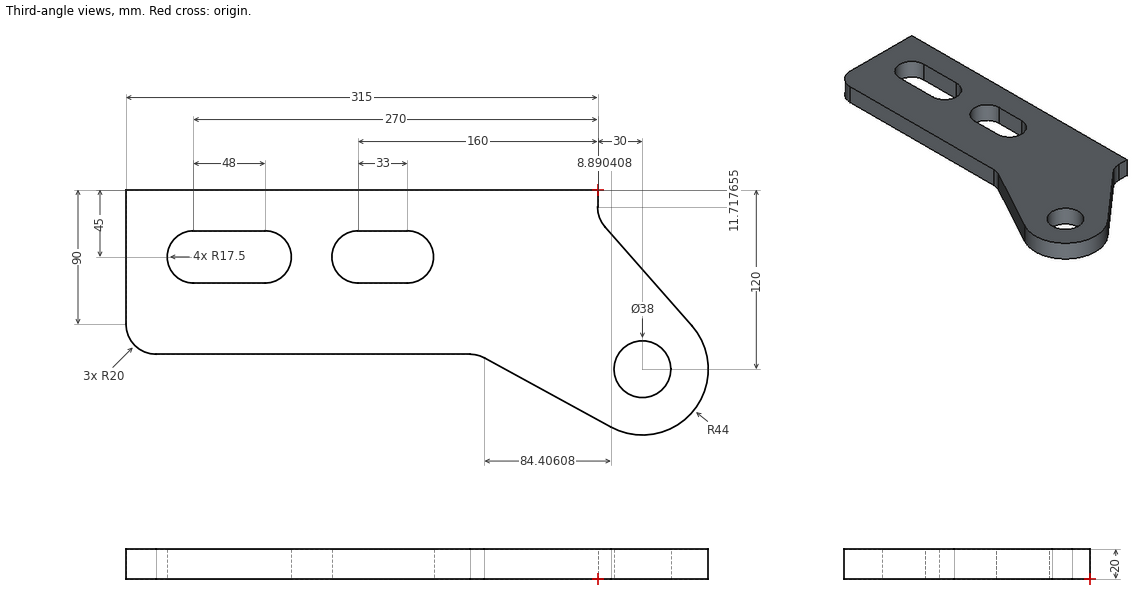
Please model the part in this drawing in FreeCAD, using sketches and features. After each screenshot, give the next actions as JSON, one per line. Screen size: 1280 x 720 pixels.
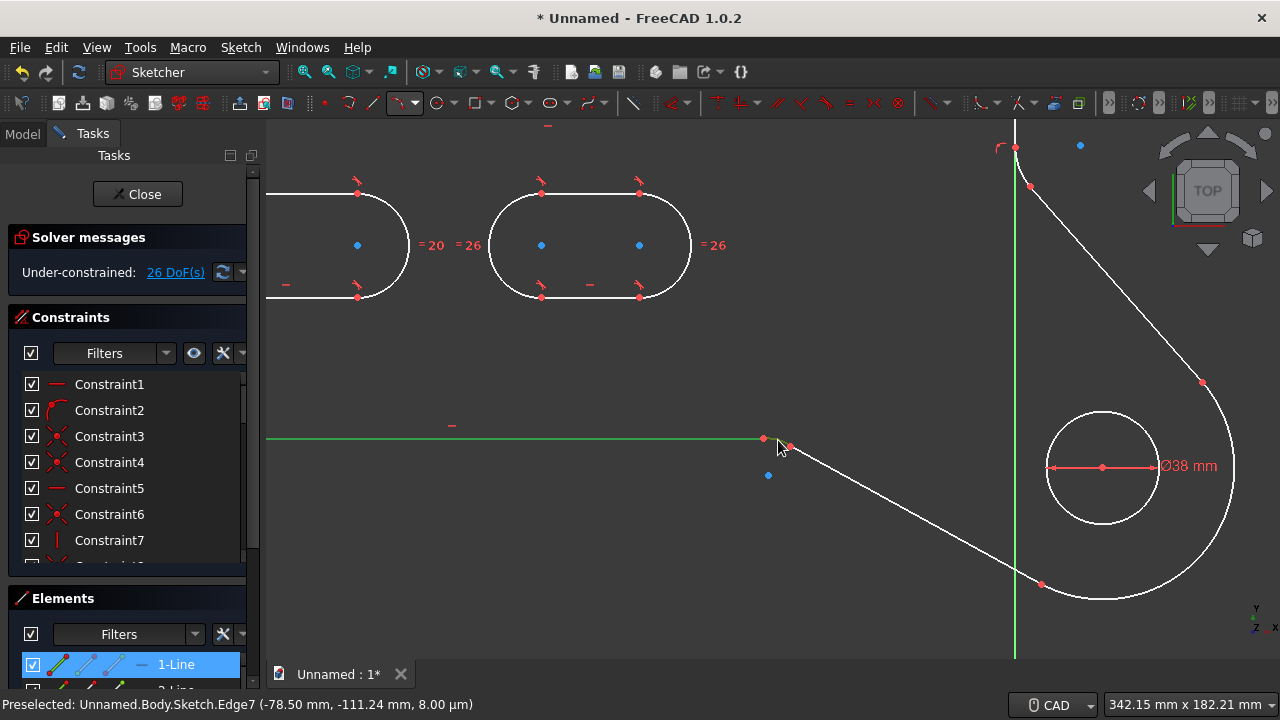
{"action": "left_click", "coordinate": [826, 104]}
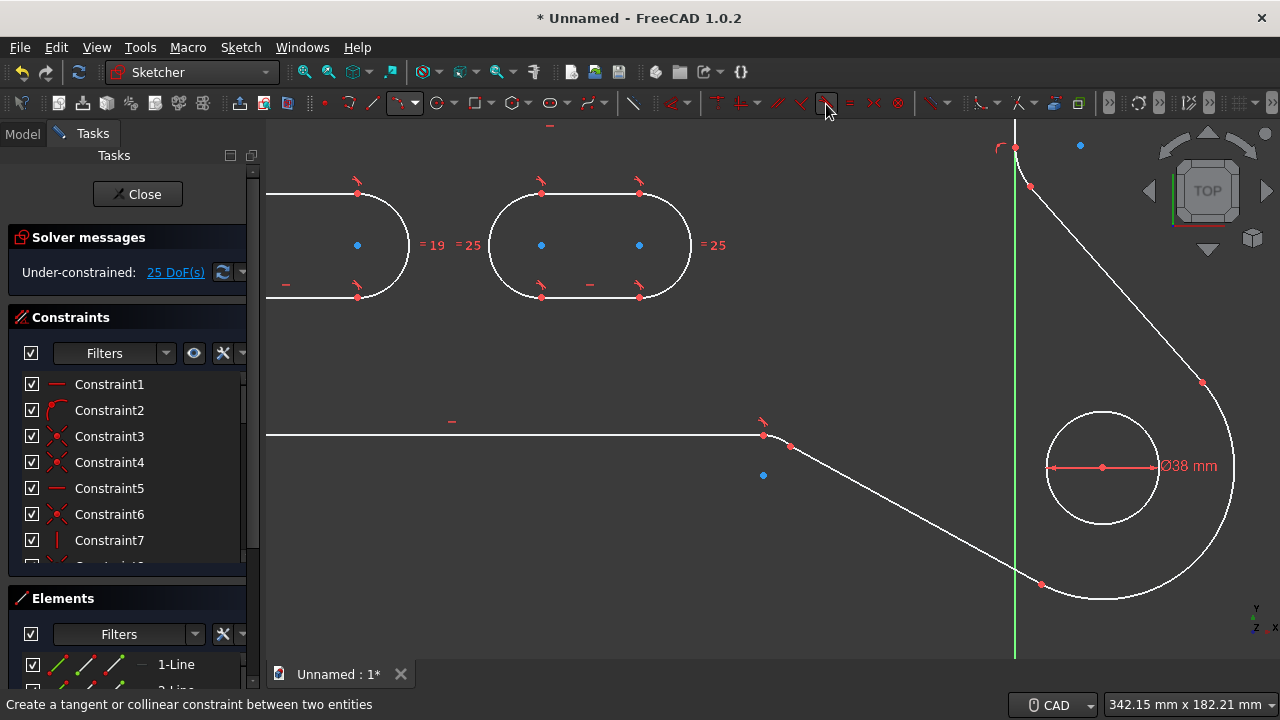
{"action": "left_click", "coordinate": [327, 435]}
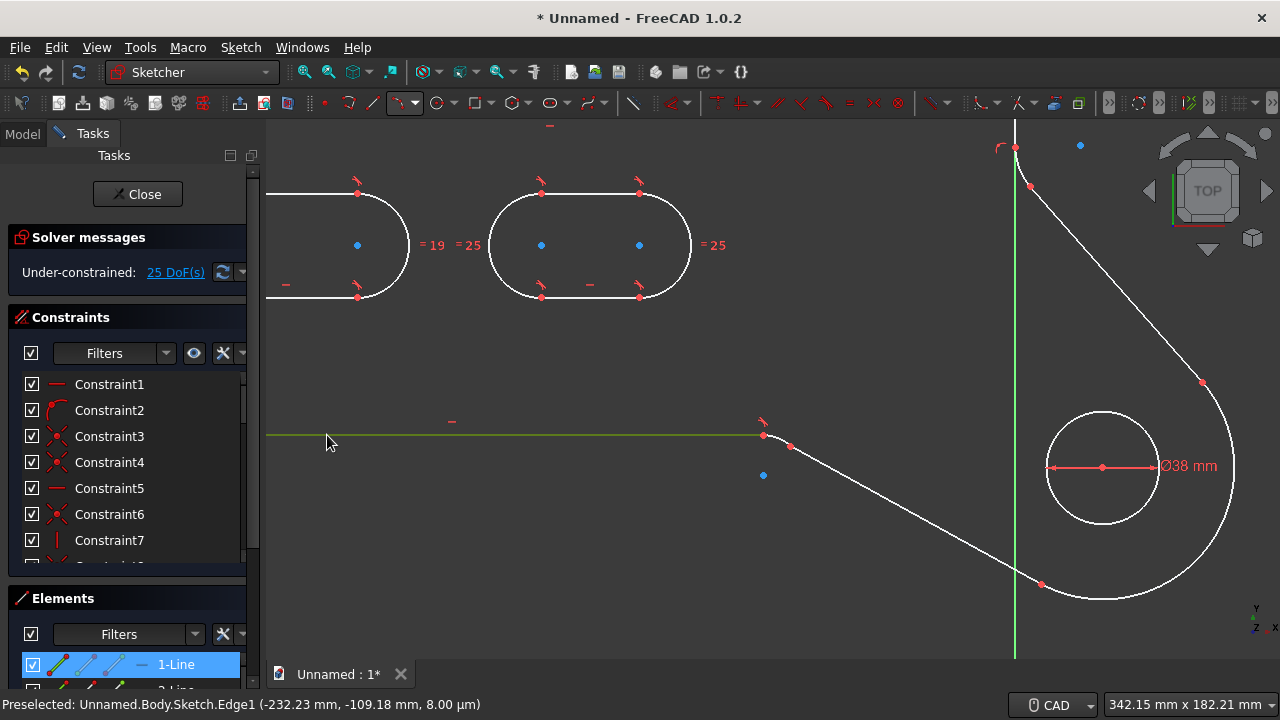
{"action": "scroll", "coordinate": [778, 440], "scroll_direction": "down", "scroll_amount": 3}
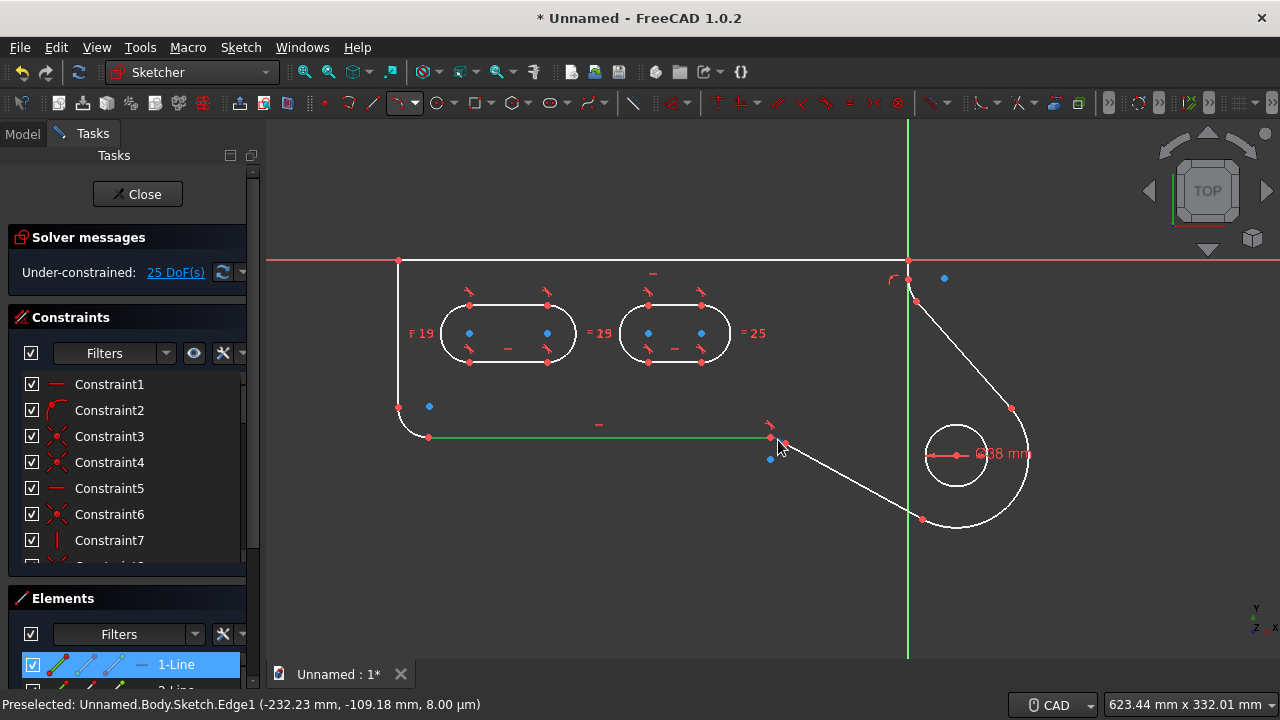
{"action": "left_click", "coordinate": [402, 421]}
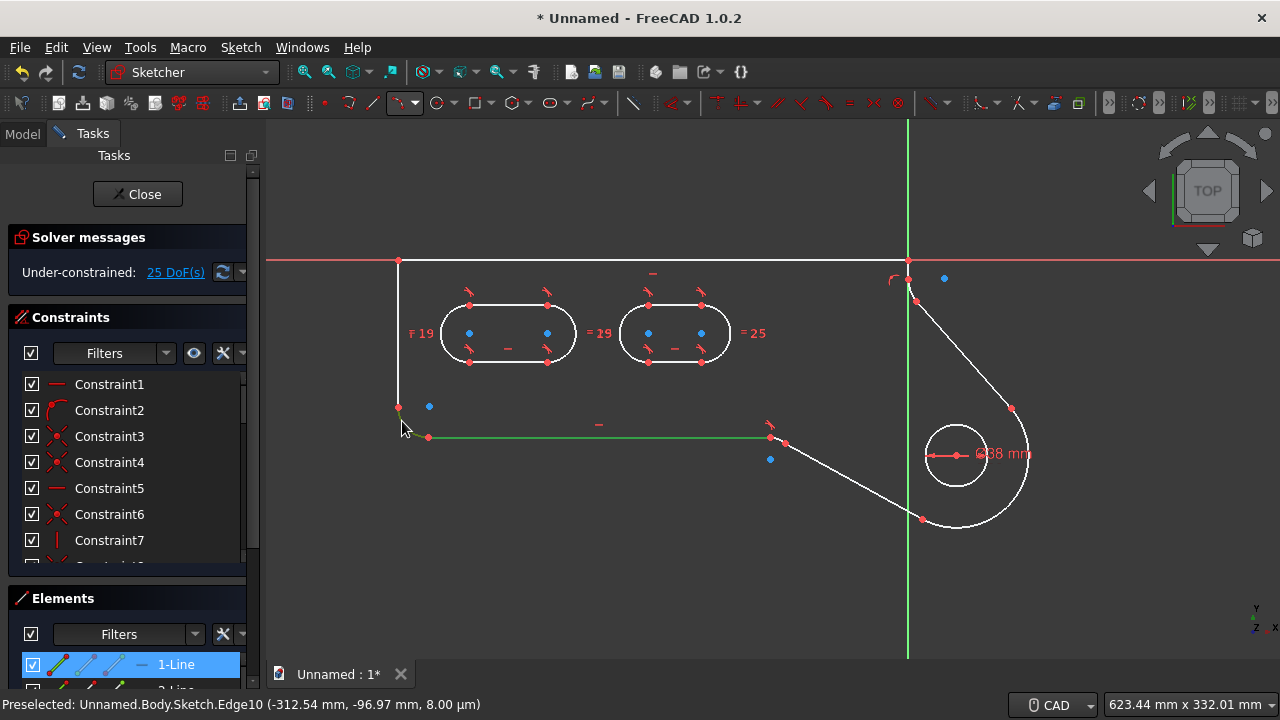
{"action": "left_click", "coordinate": [826, 104]}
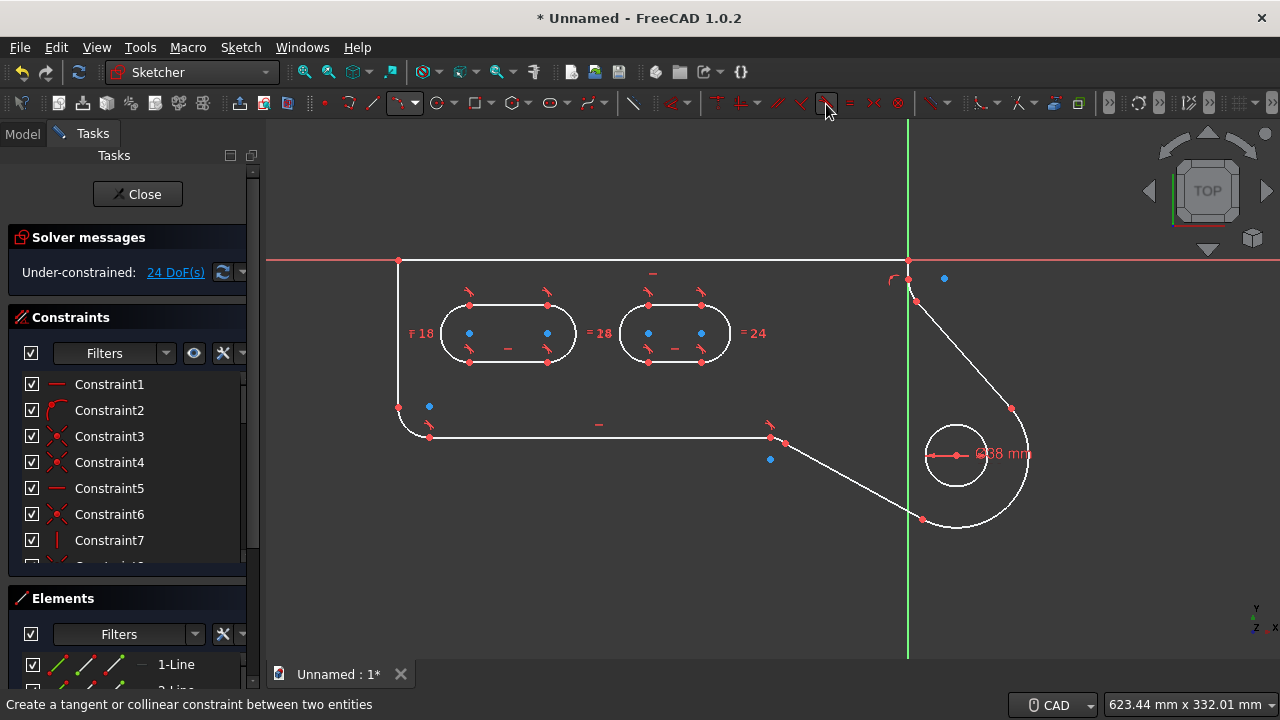
{"action": "left_click", "coordinate": [826, 466]}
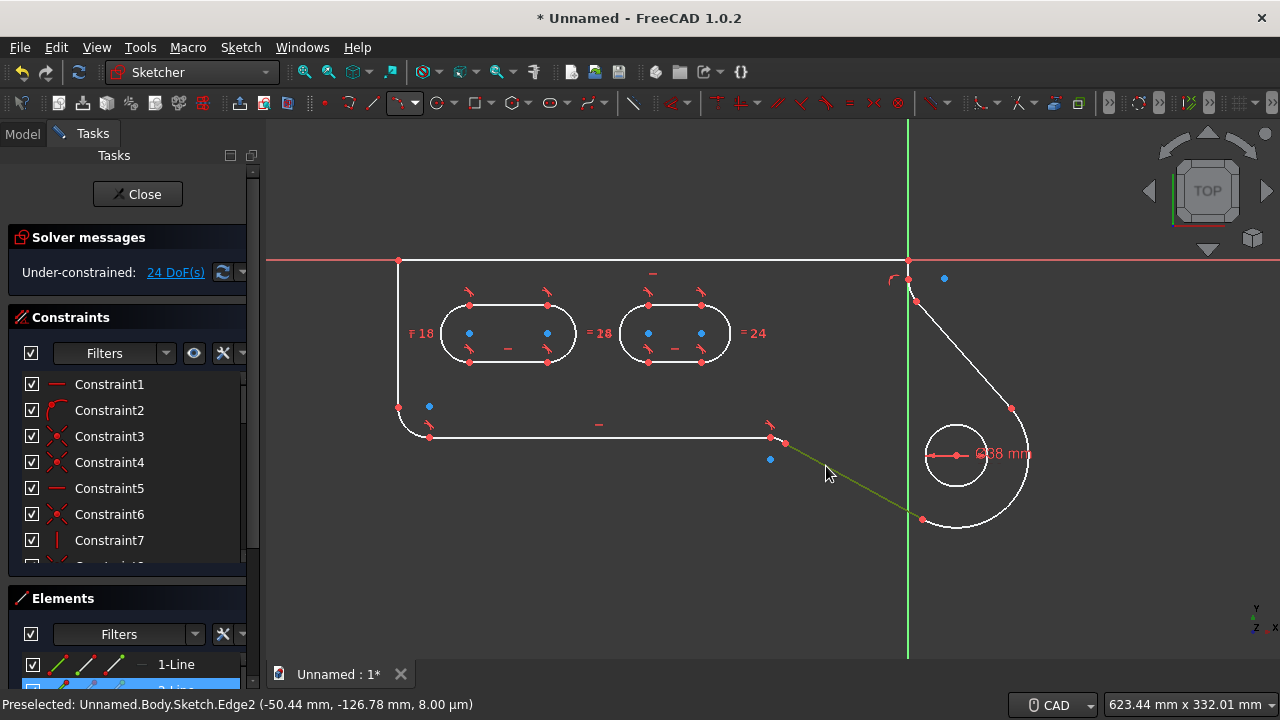
{"action": "scroll", "coordinate": [778, 439], "scroll_direction": "up", "scroll_amount": 3}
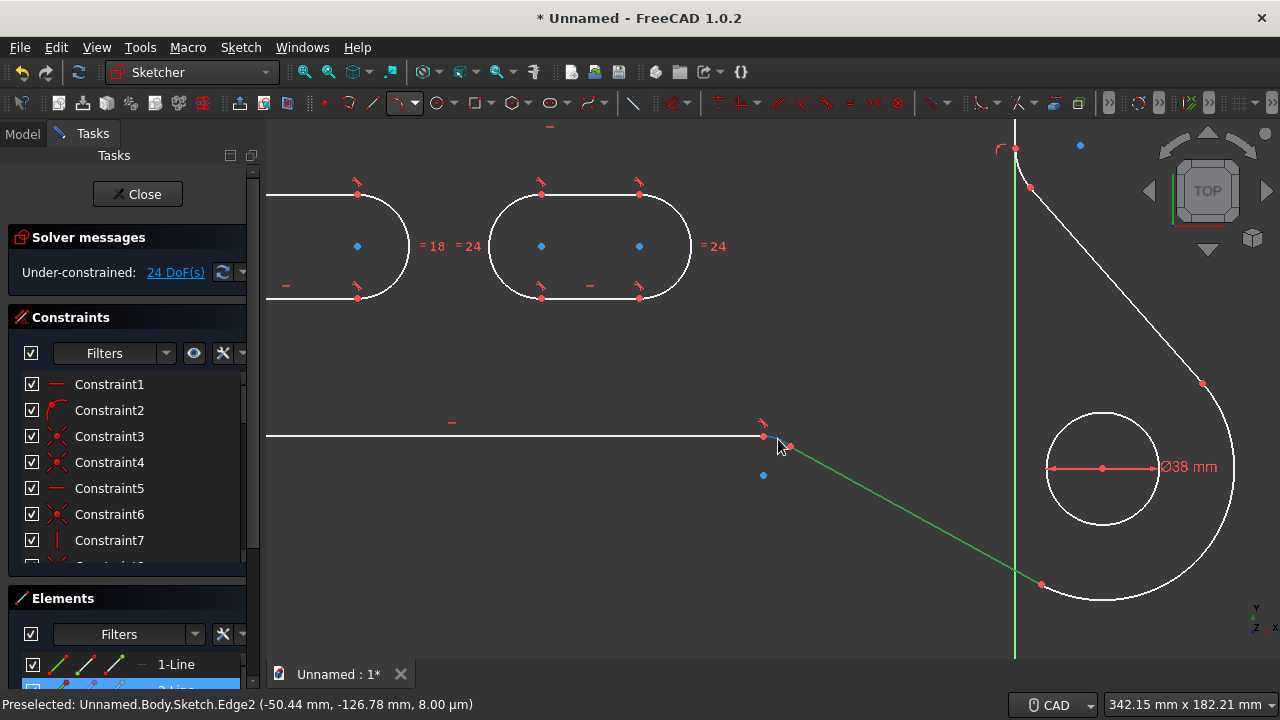
{"action": "left_click", "coordinate": [778, 439]}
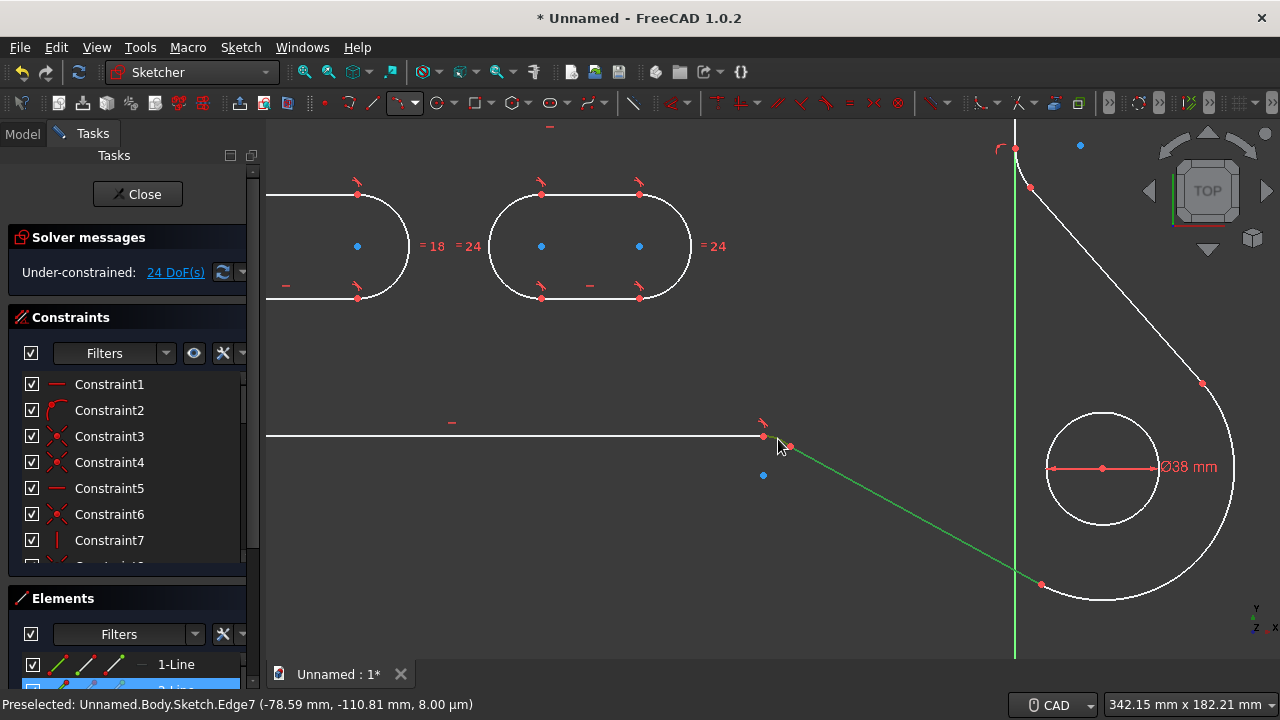
{"action": "left_click", "coordinate": [826, 104]}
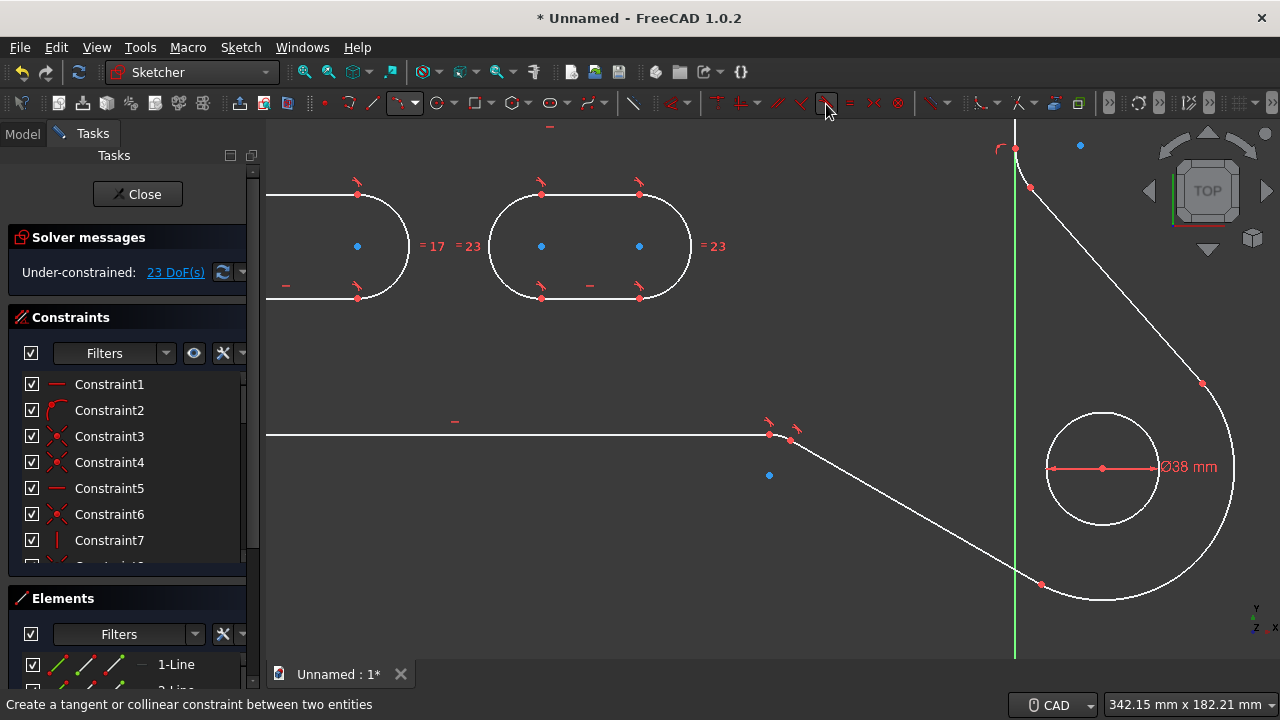
{"action": "left_click", "coordinate": [1082, 246]}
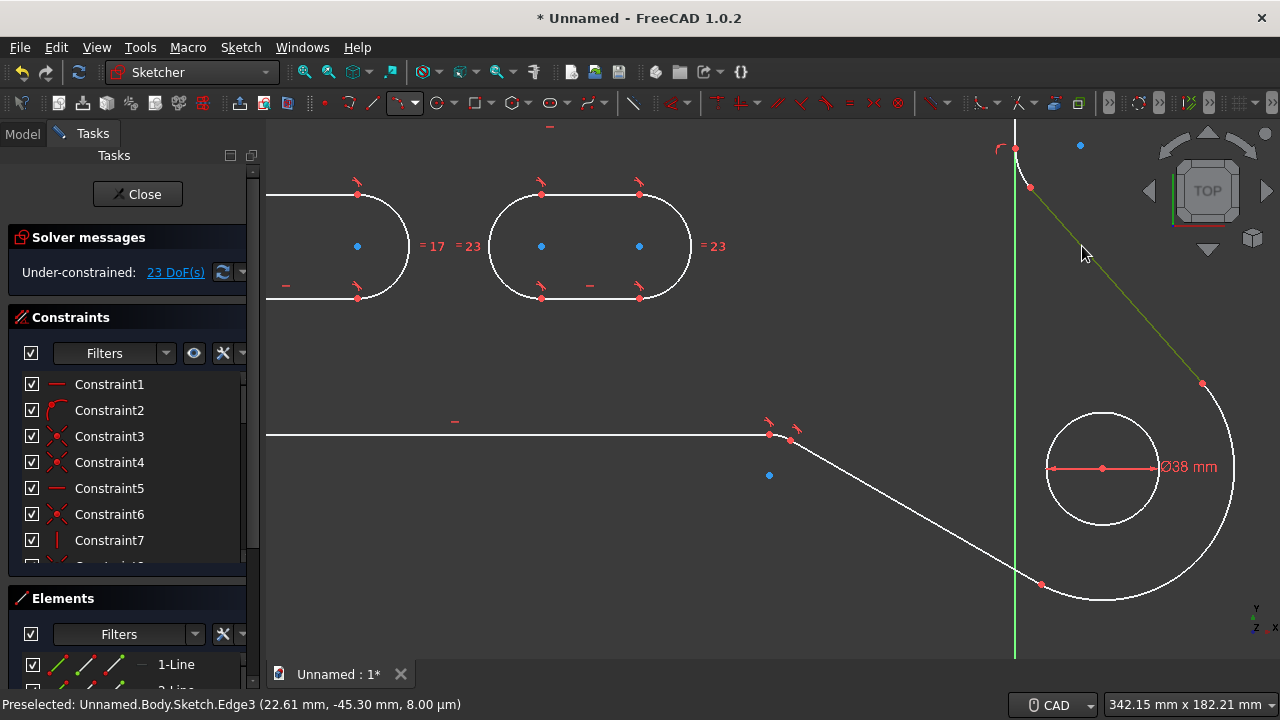
{"action": "left_click", "coordinate": [1111, 600]}